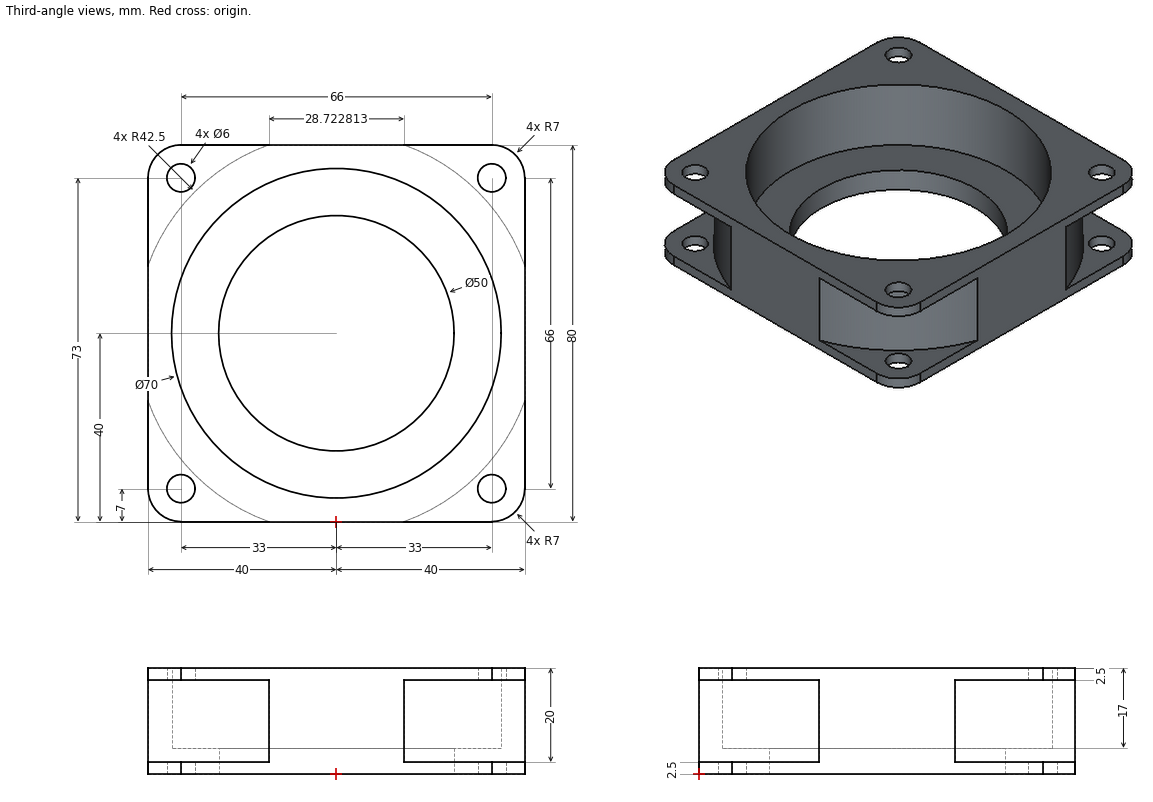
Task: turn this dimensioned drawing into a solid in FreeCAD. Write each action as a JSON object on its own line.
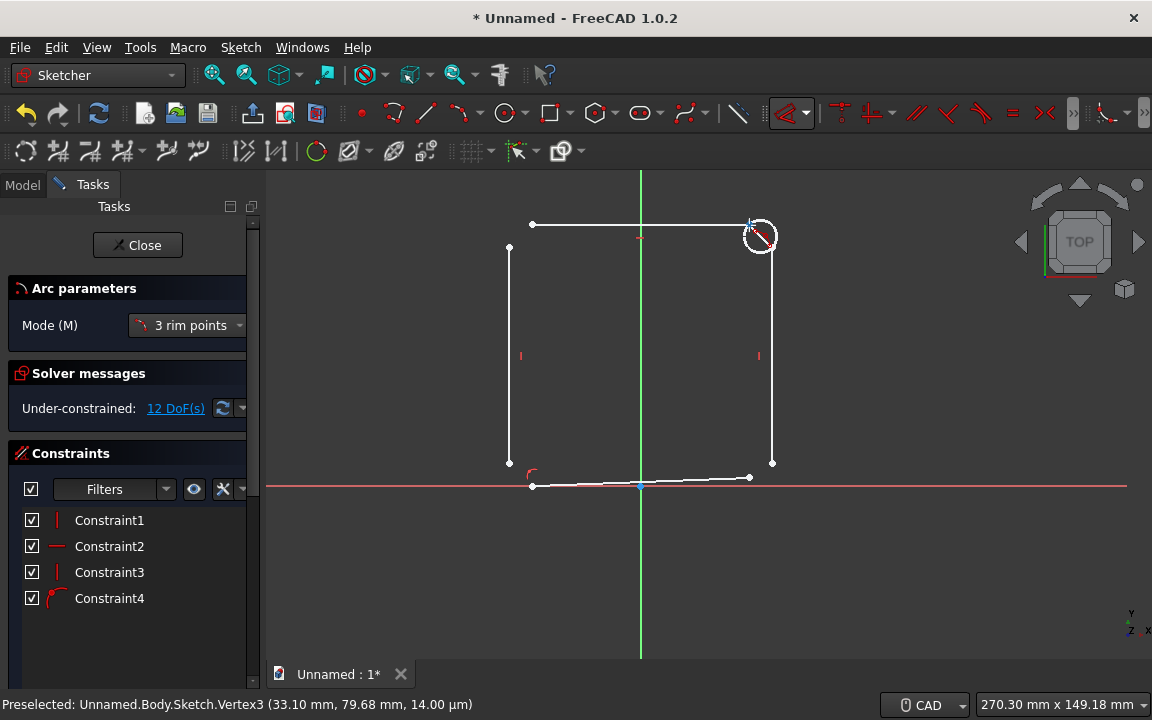
{"action": "scroll", "coordinate": [765, 231], "scroll_direction": "up", "scroll_amount": 5}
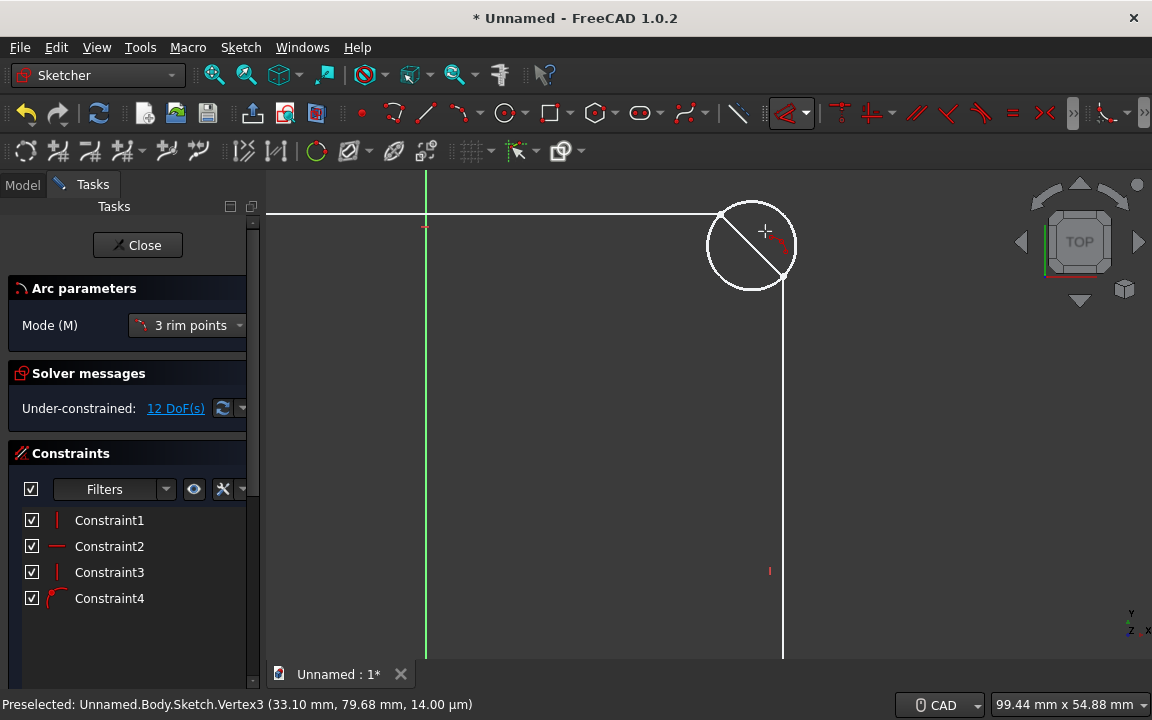
{"action": "left_click", "coordinate": [764, 230]}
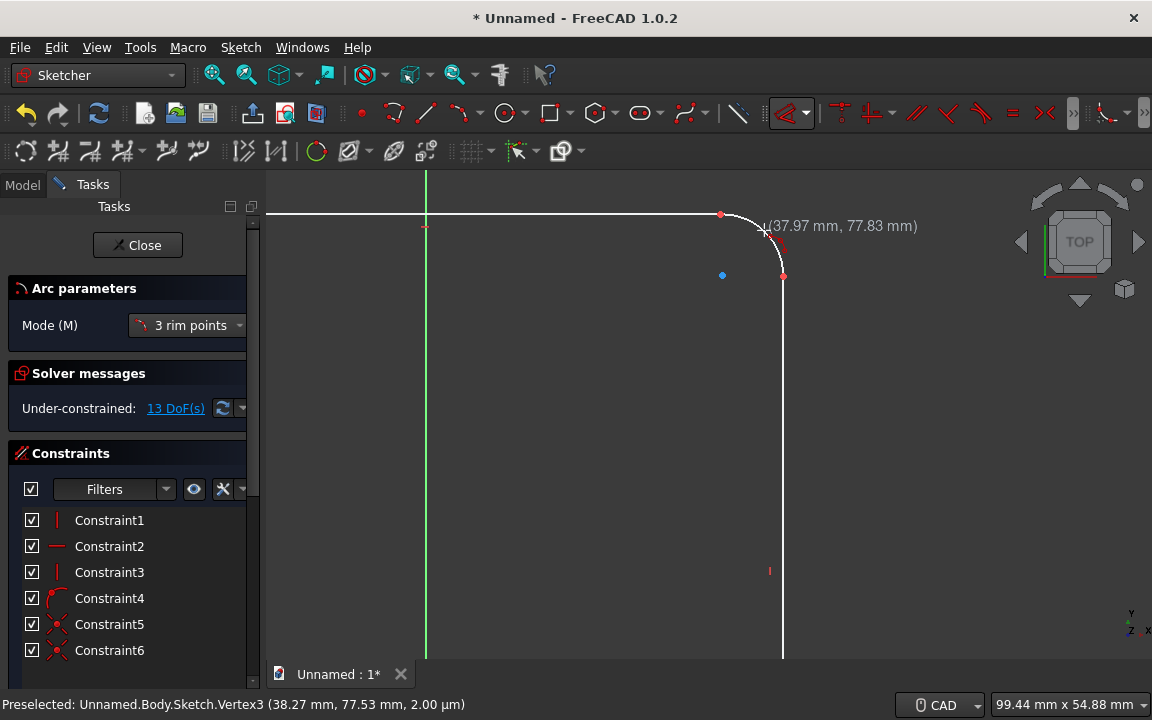
{"action": "scroll", "coordinate": [816, 289], "scroll_direction": "down", "scroll_amount": 4}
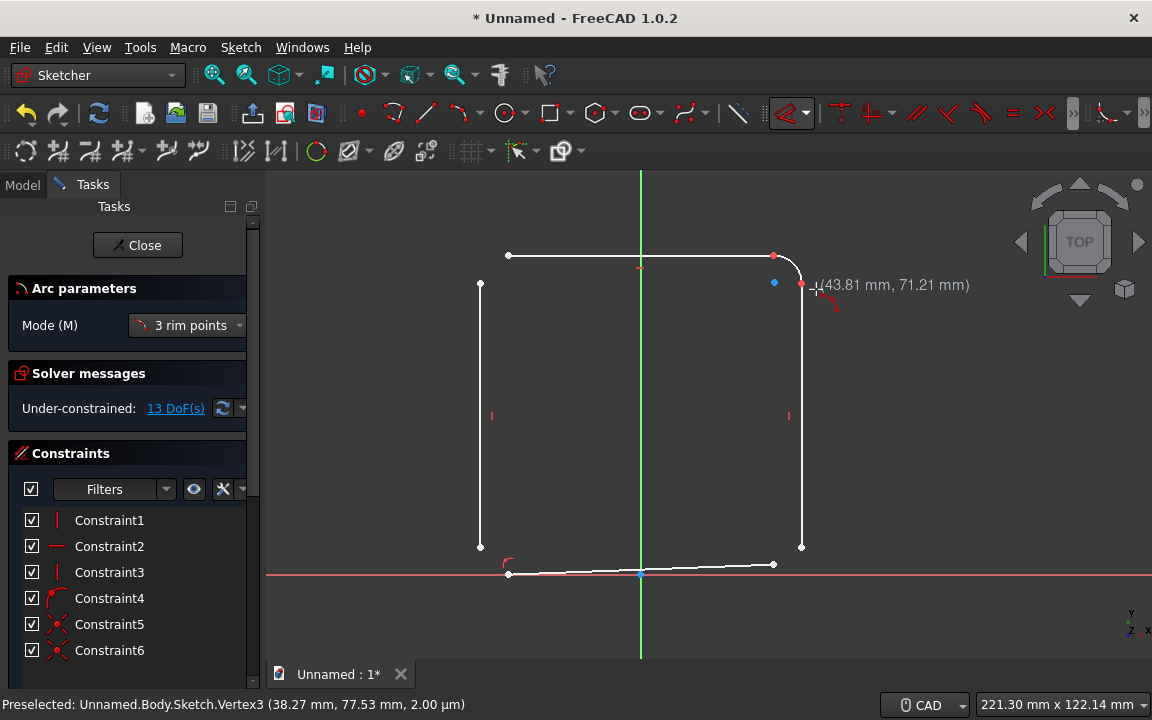
{"action": "left_click", "coordinate": [508, 256]}
{"action": "left_click", "coordinate": [480, 284]}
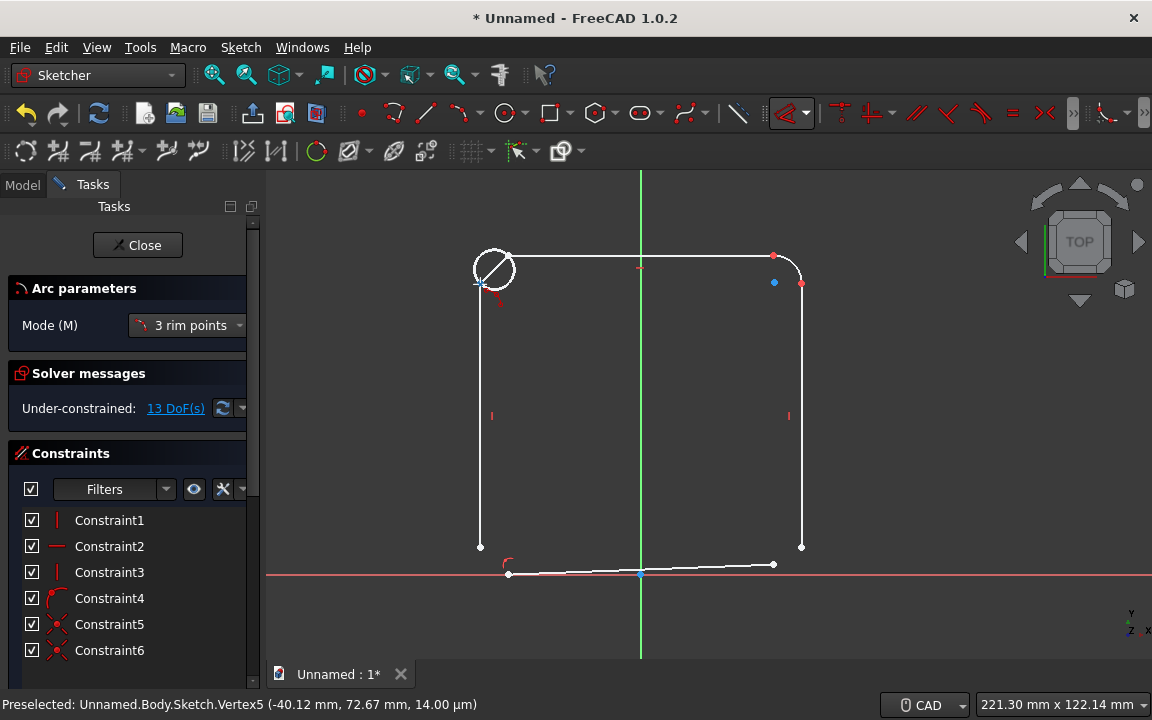
{"action": "scroll", "coordinate": [489, 263], "scroll_direction": "up", "scroll_amount": 4}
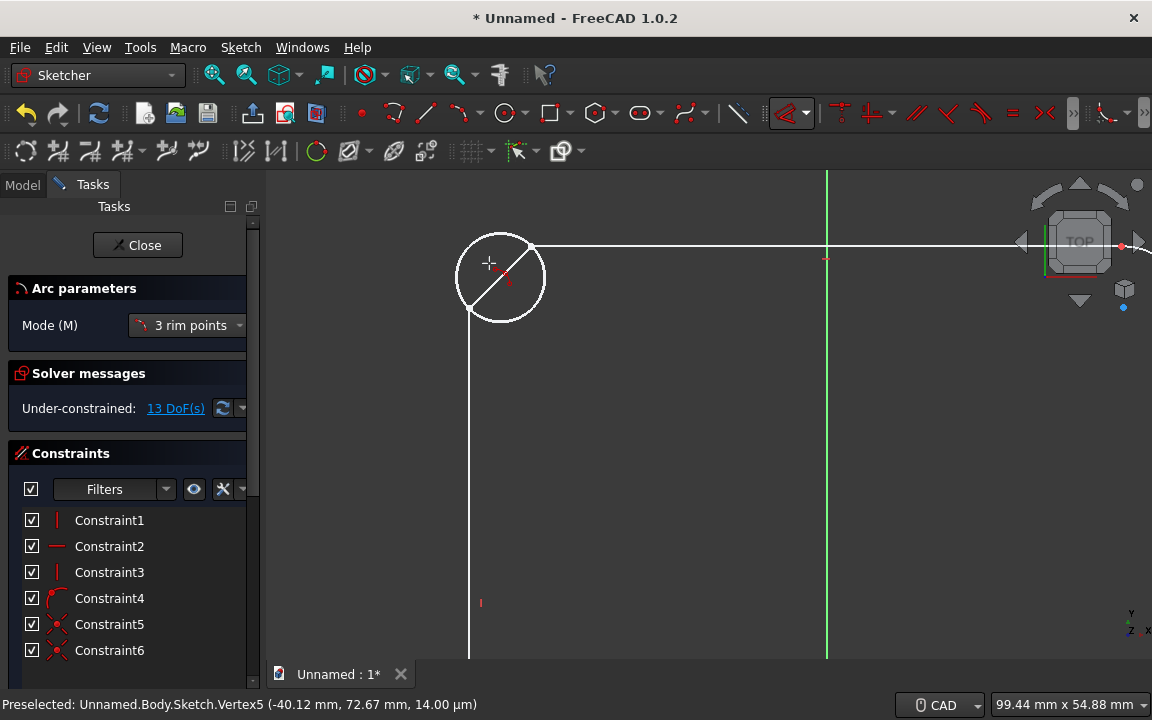
{"action": "left_click", "coordinate": [489, 262]}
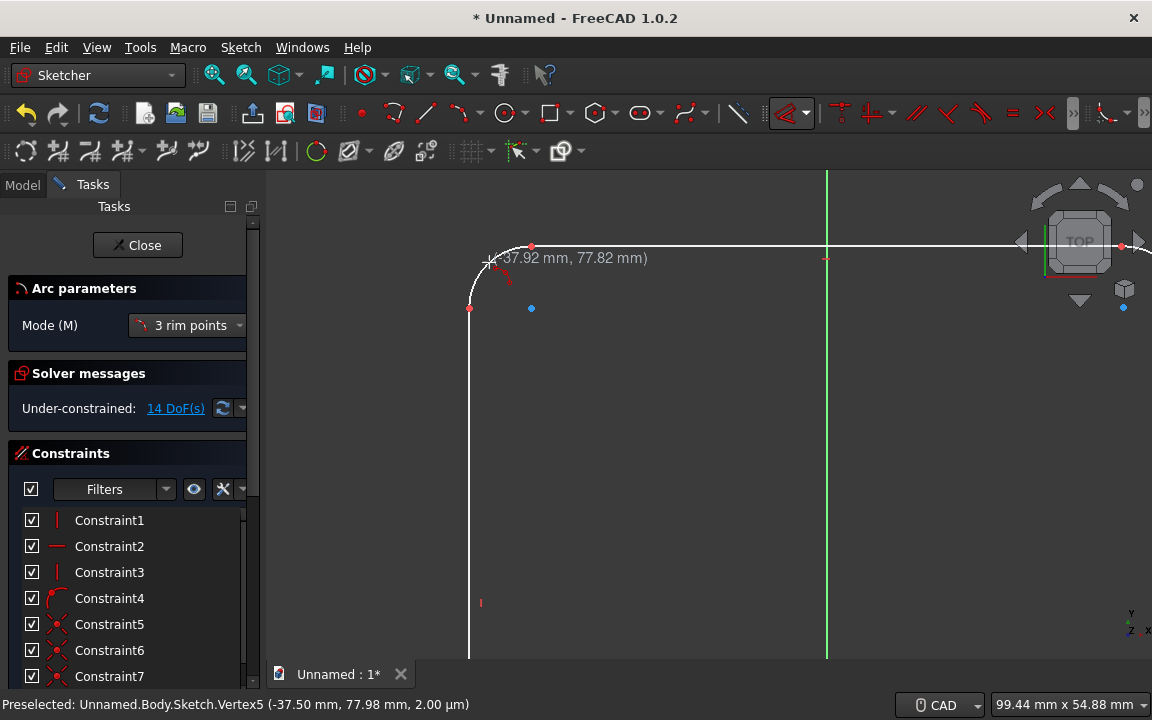
{"action": "scroll", "coordinate": [488, 263], "scroll_direction": "down", "scroll_amount": 4}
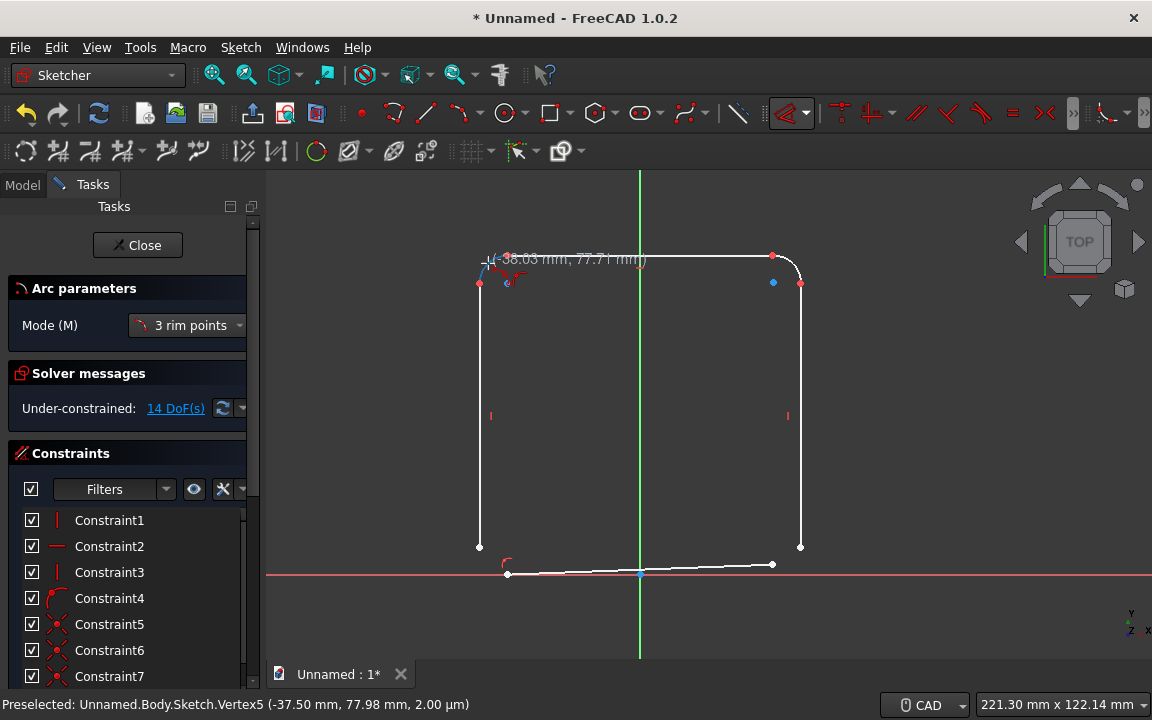
{"action": "left_click", "coordinate": [480, 548]}
{"action": "left_click", "coordinate": [508, 575]}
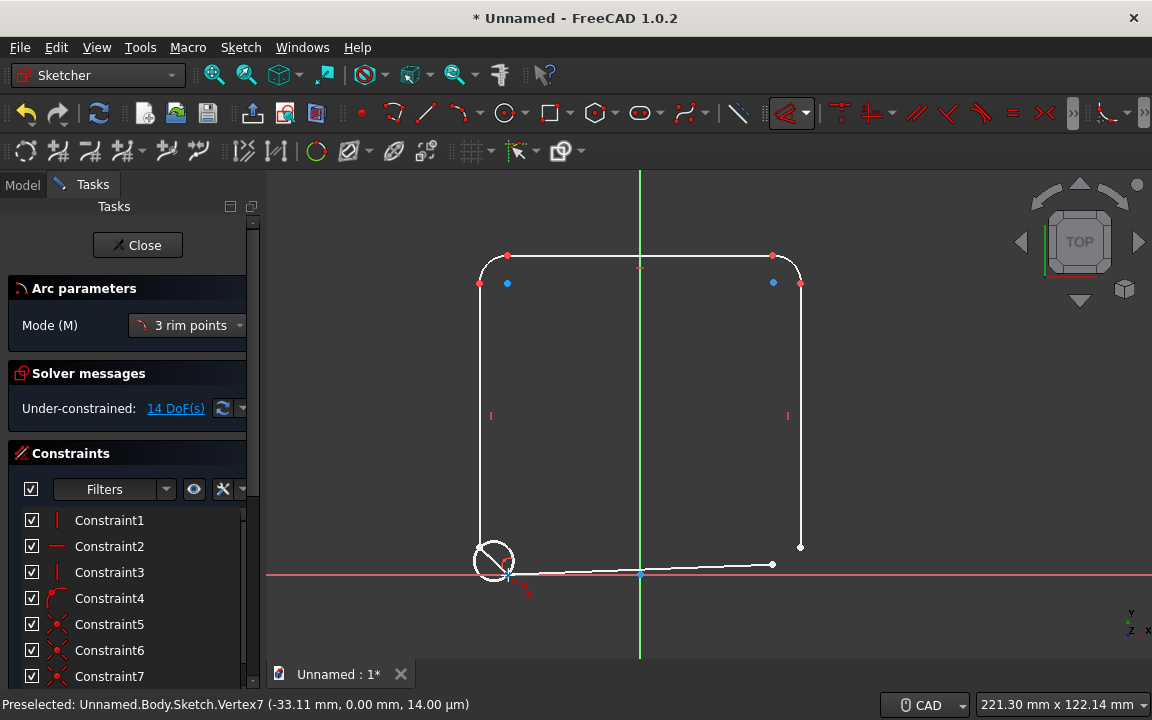
{"action": "scroll", "coordinate": [488, 566], "scroll_direction": "up", "scroll_amount": 4}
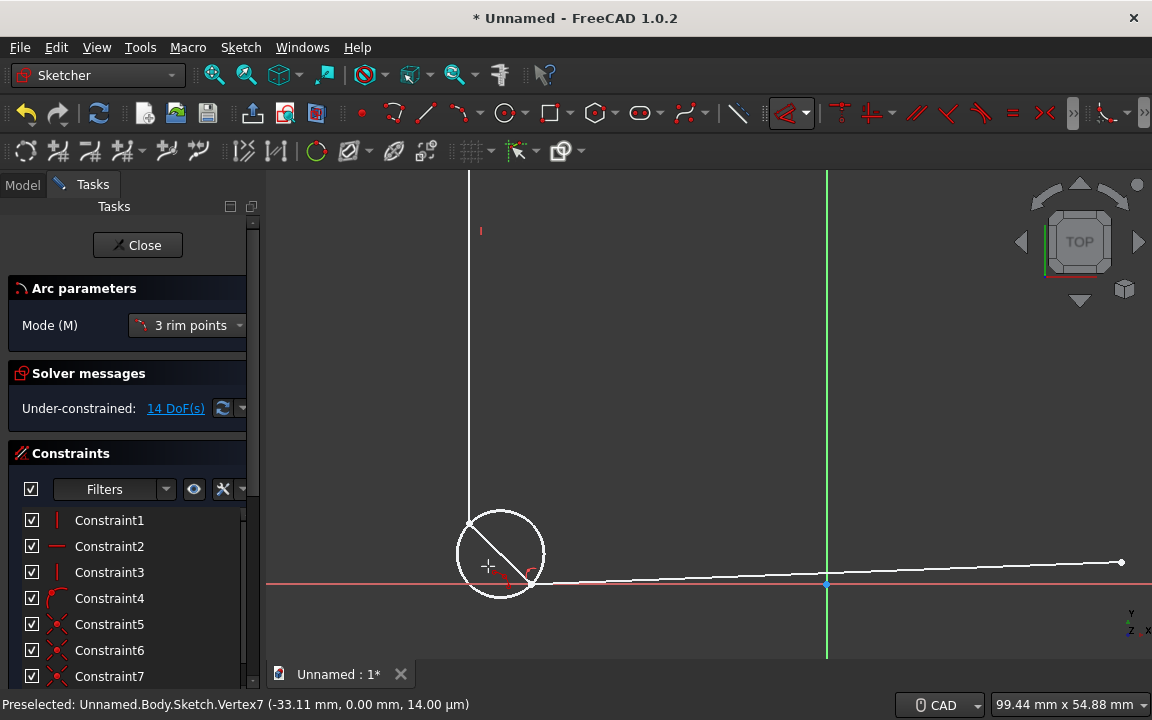
{"action": "left_click", "coordinate": [489, 566]}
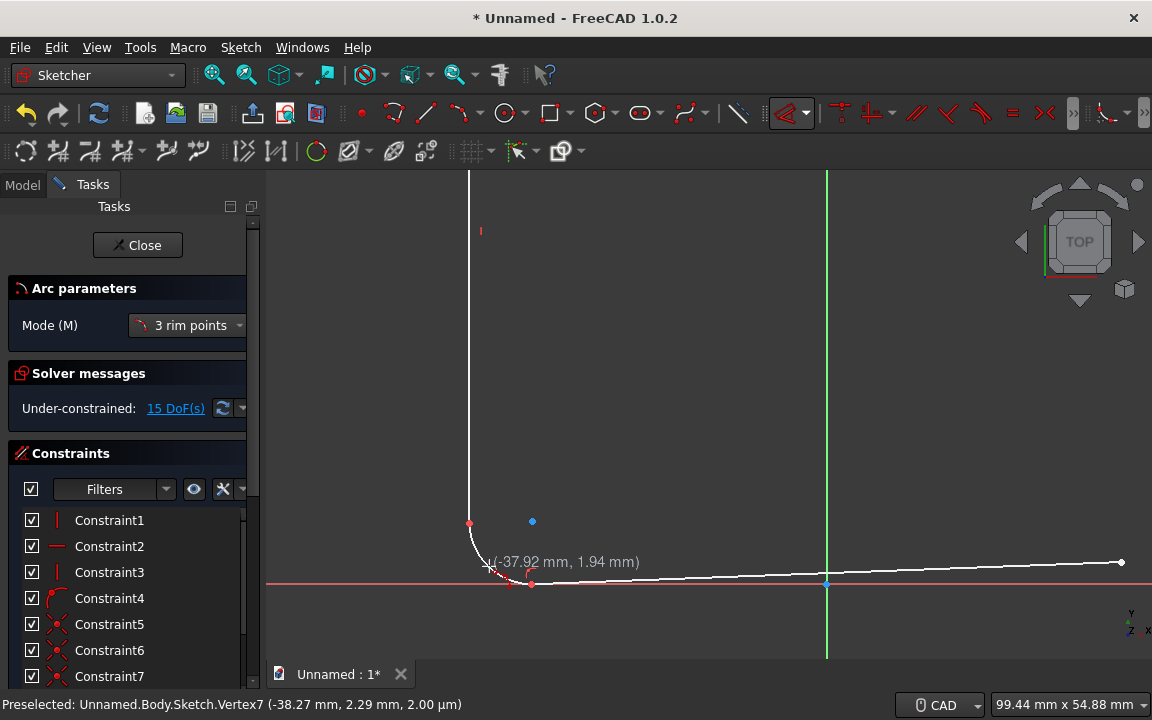
{"action": "scroll", "coordinate": [488, 567], "scroll_direction": "down", "scroll_amount": 4}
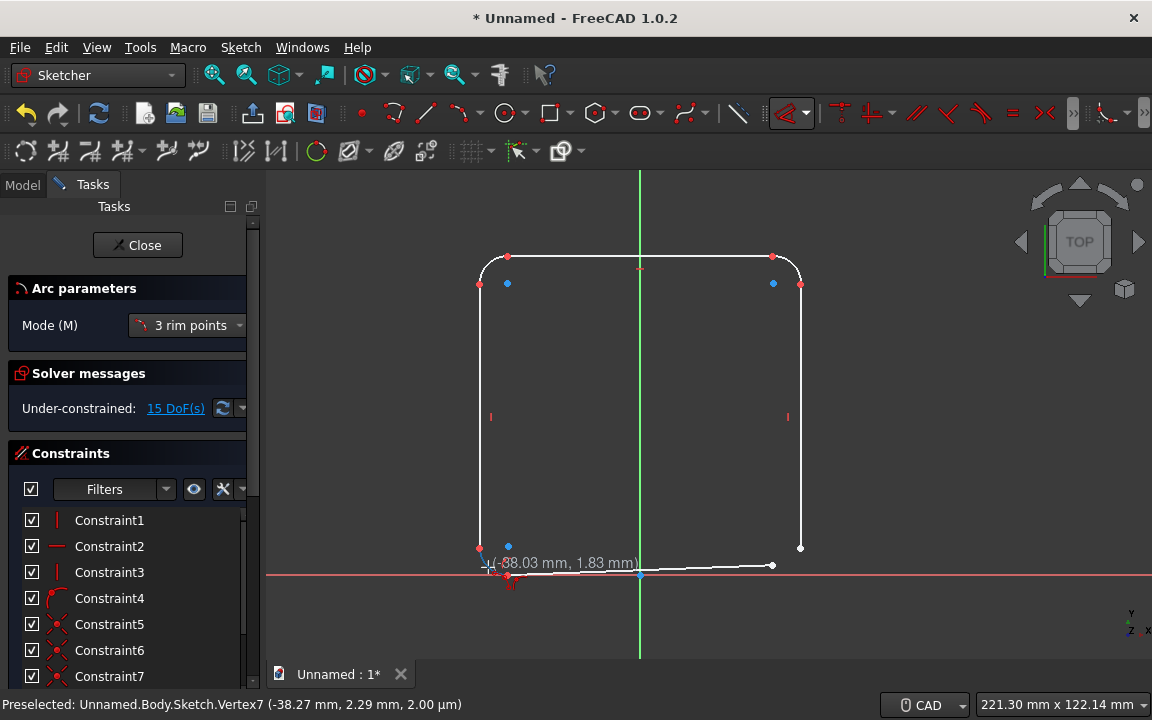
{"action": "left_click", "coordinate": [773, 565]}
{"action": "left_click", "coordinate": [801, 548]}